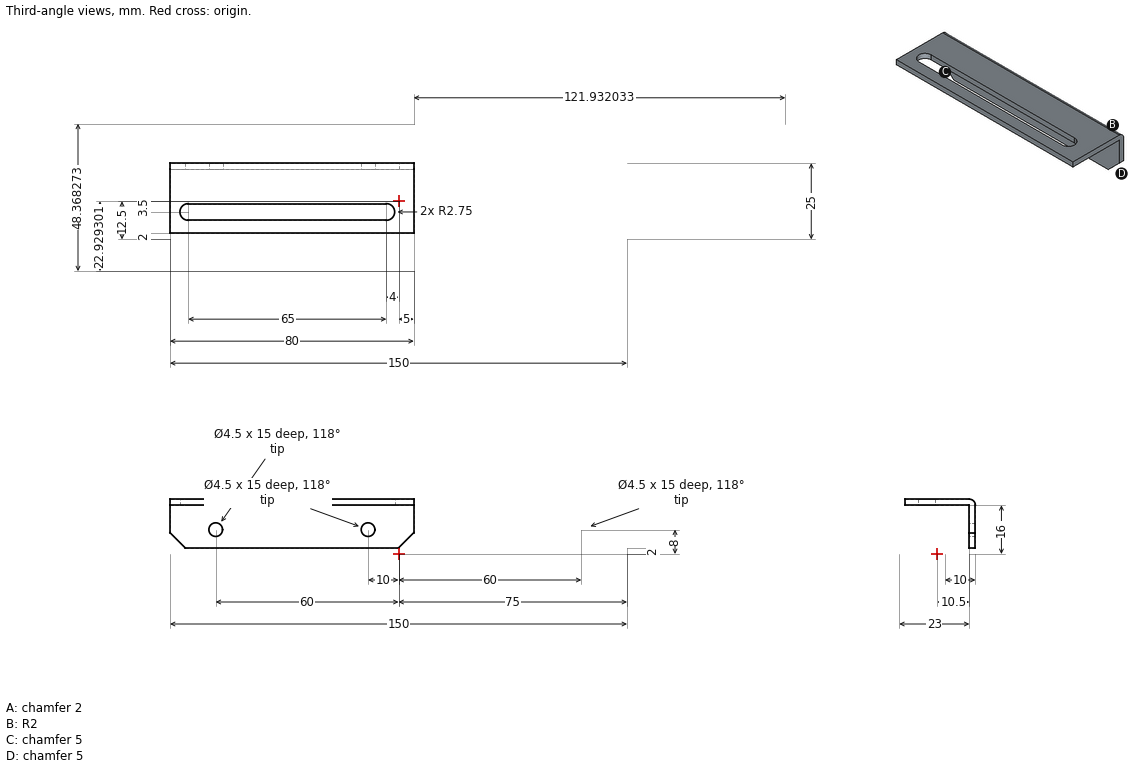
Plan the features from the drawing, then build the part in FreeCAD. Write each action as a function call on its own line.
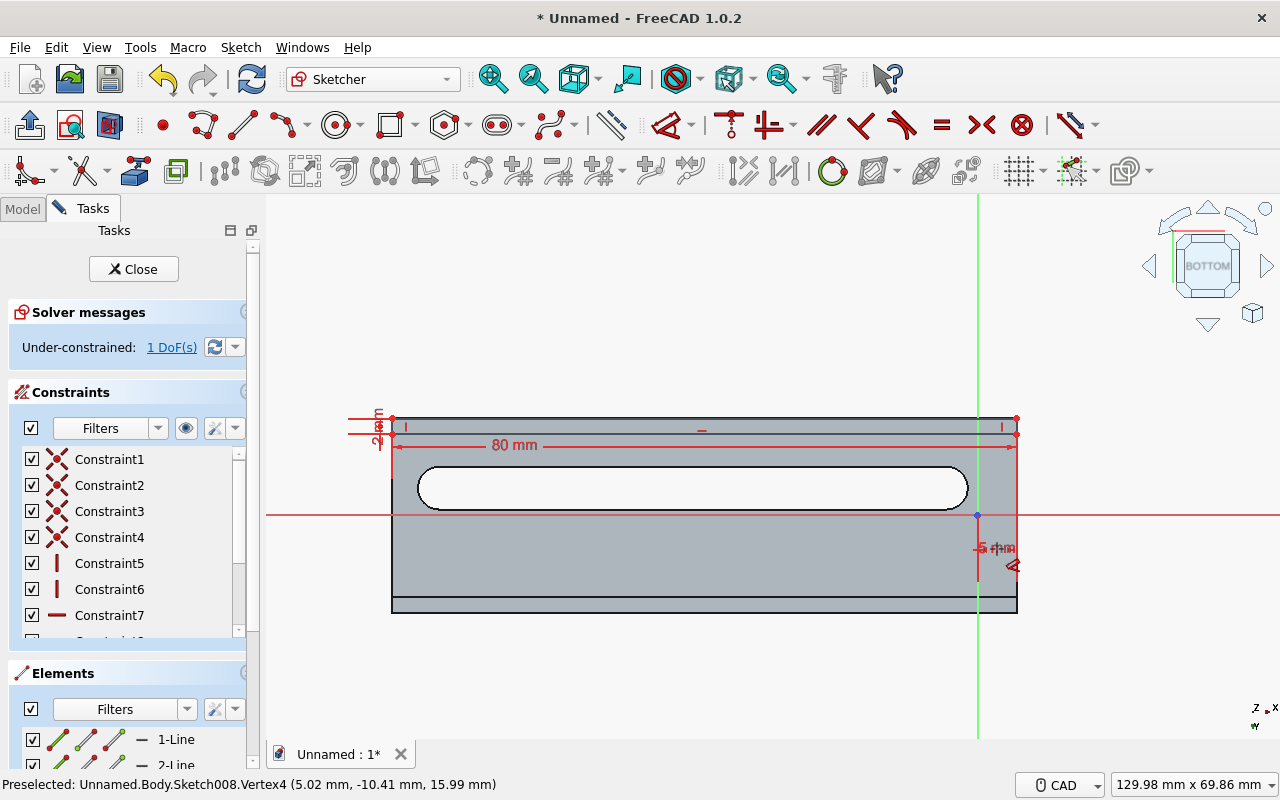
click(392, 419)
click(358, 467)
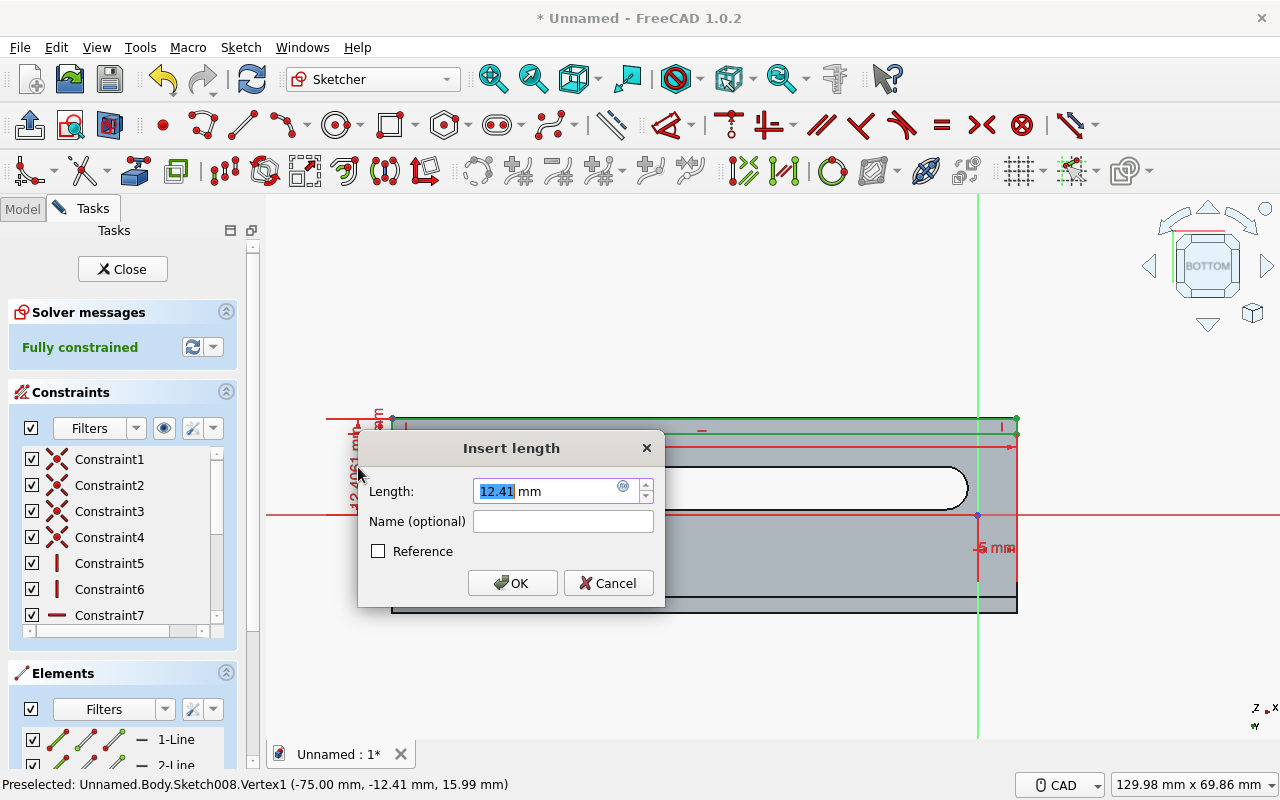
text(12.5)
key(Return)
key(Escape)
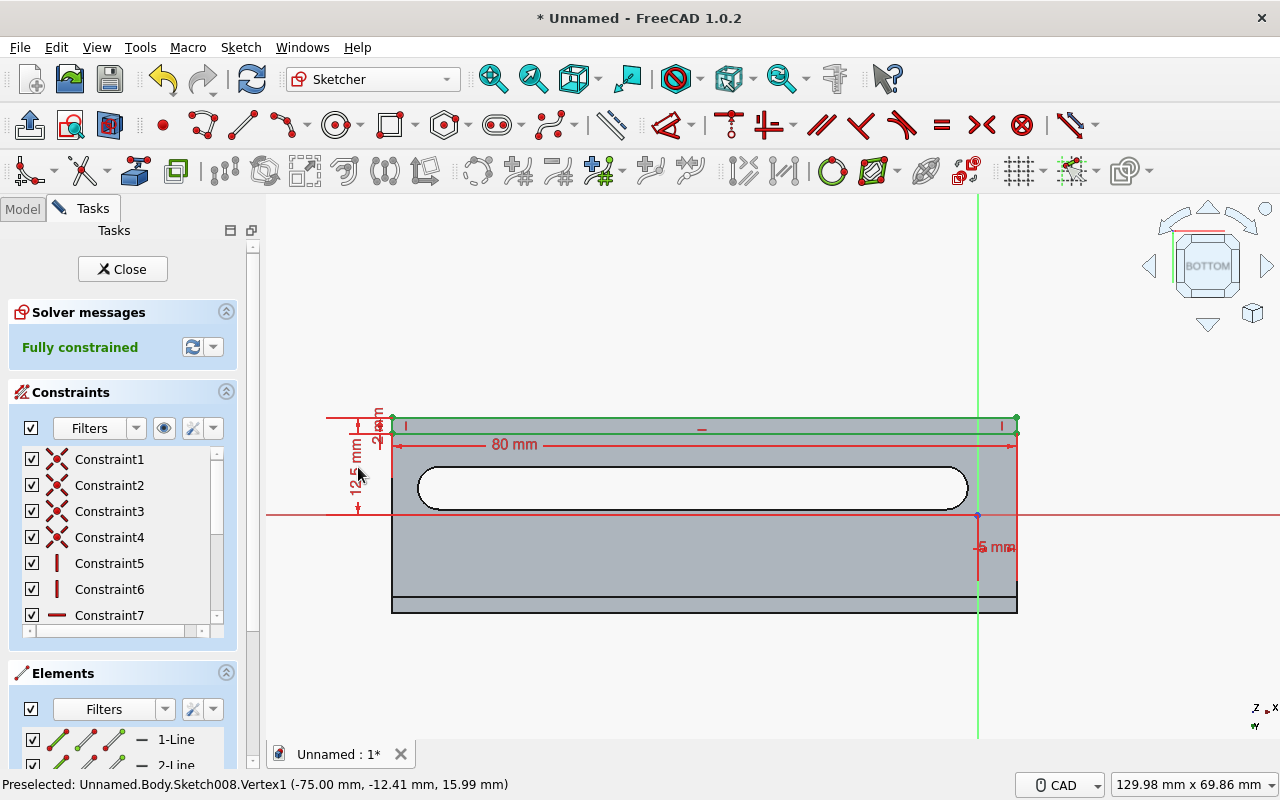
click(123, 269)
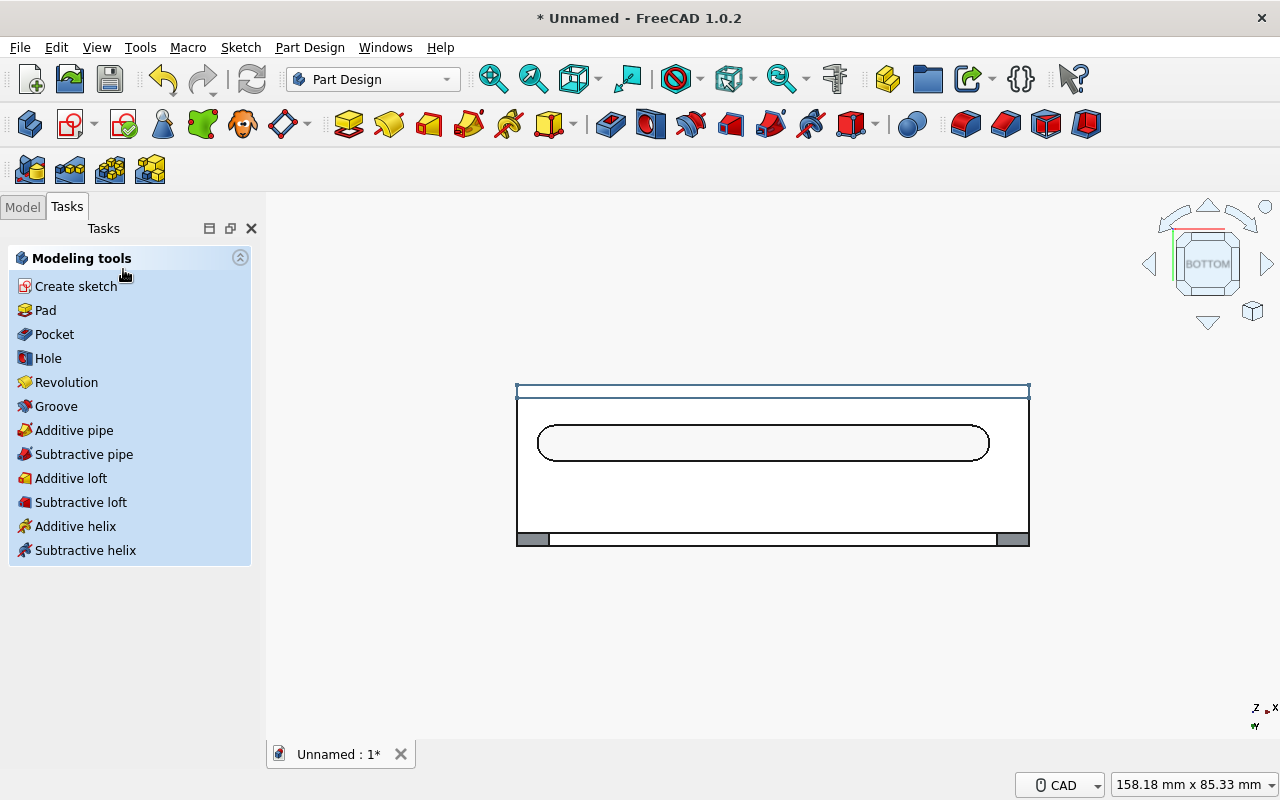
click(612, 124)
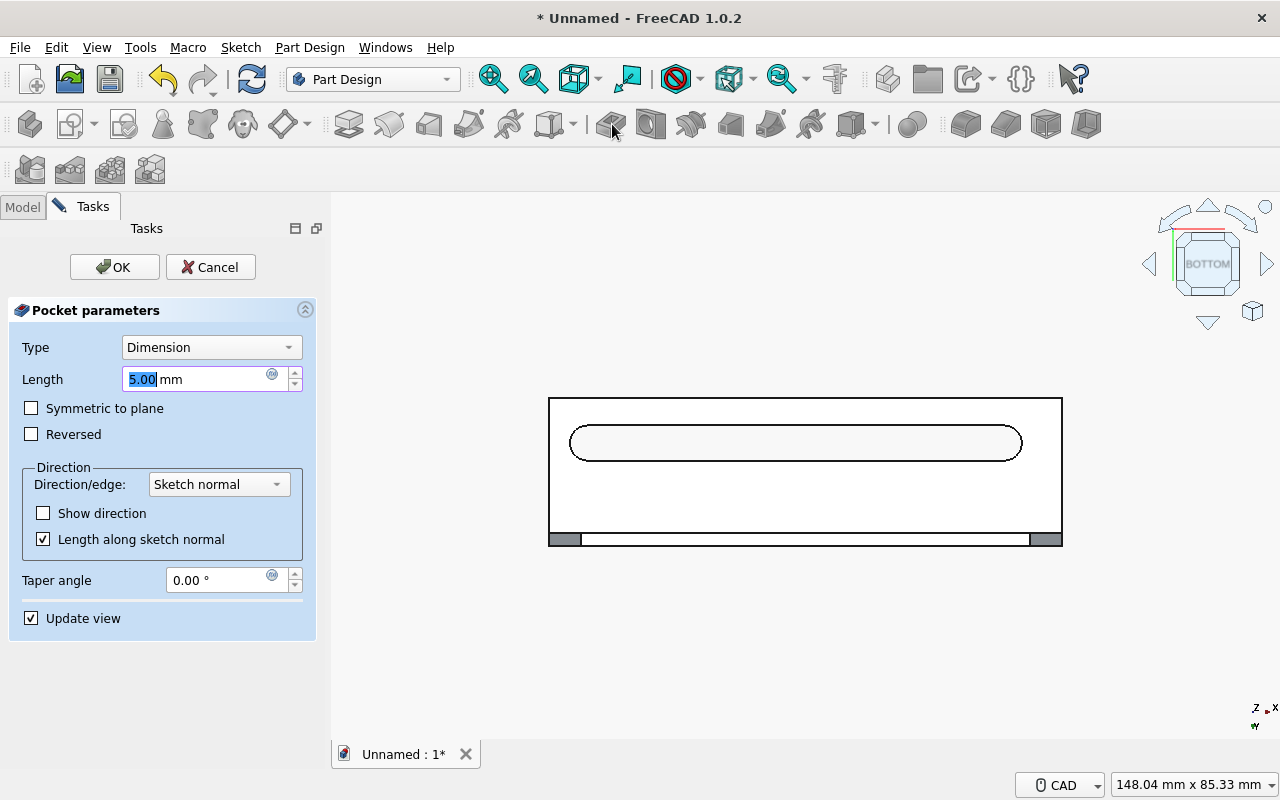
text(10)
key(Tab)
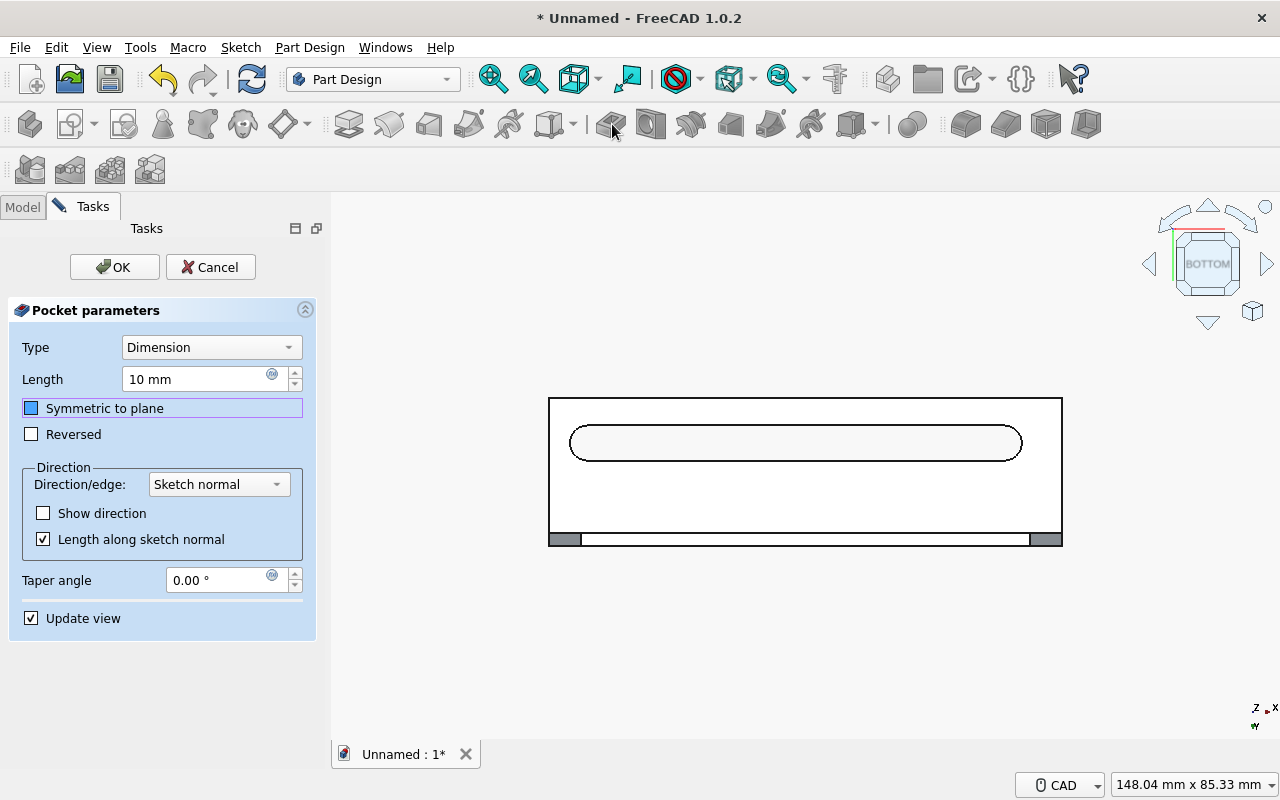
click(115, 267)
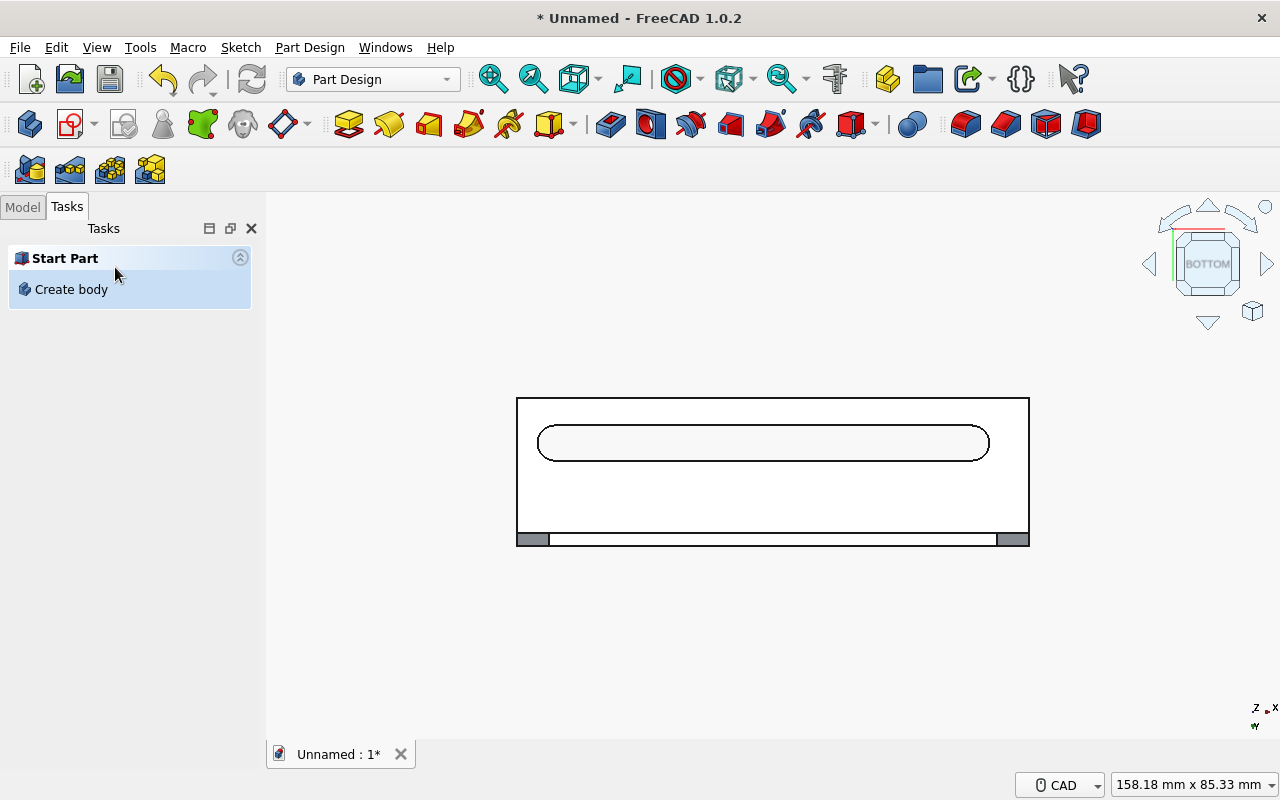
key(0)